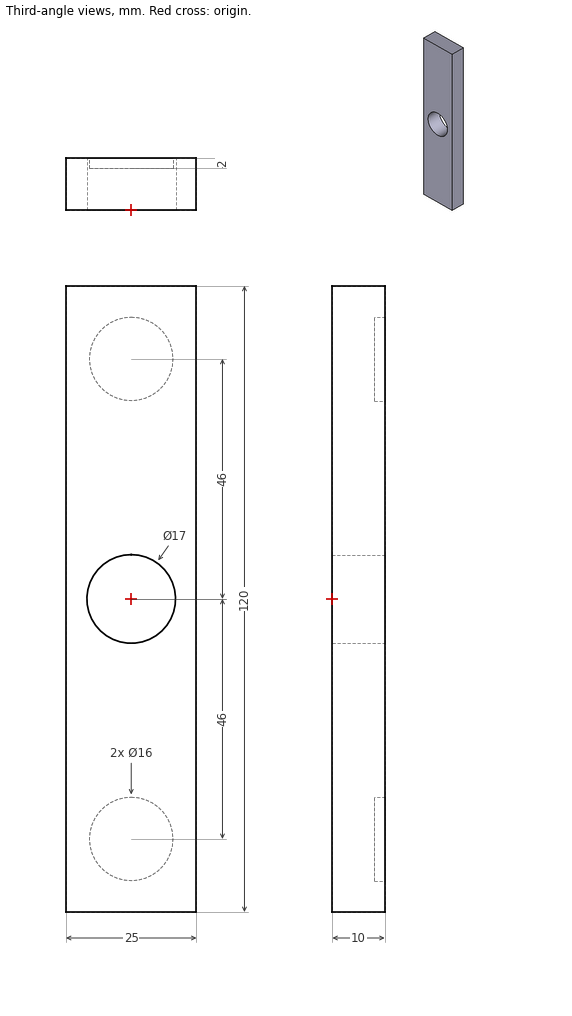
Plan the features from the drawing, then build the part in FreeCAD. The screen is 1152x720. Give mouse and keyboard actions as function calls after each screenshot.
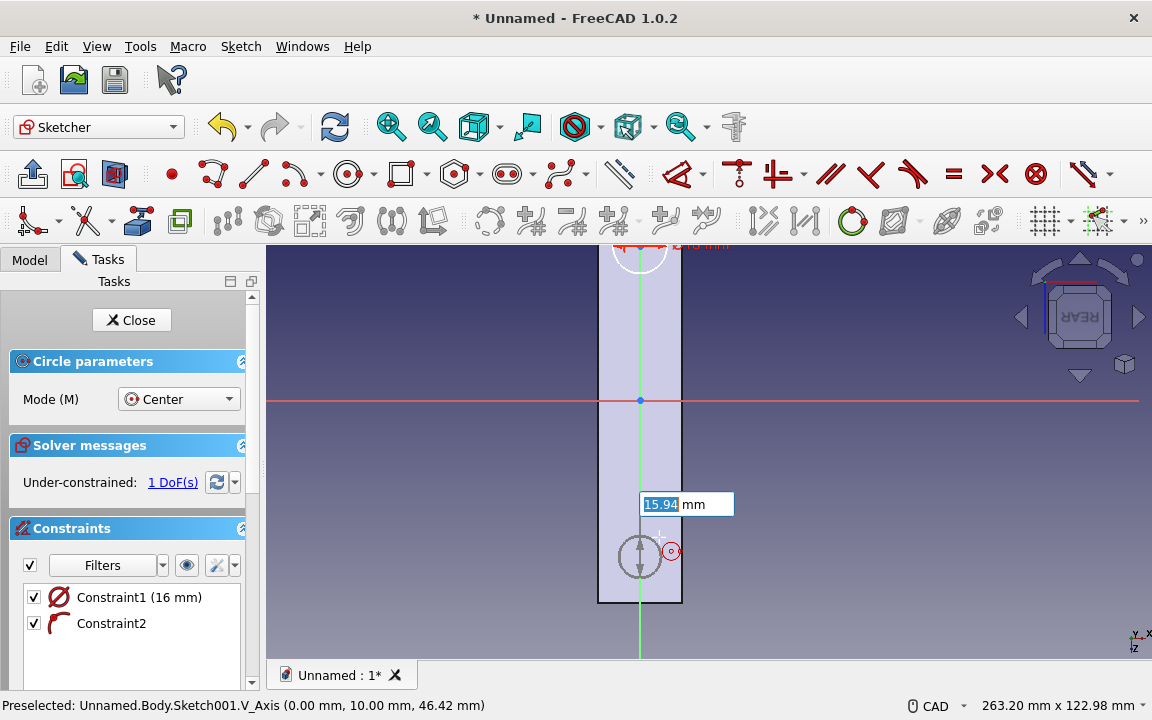
text(16)
key(Return)
key(Escape)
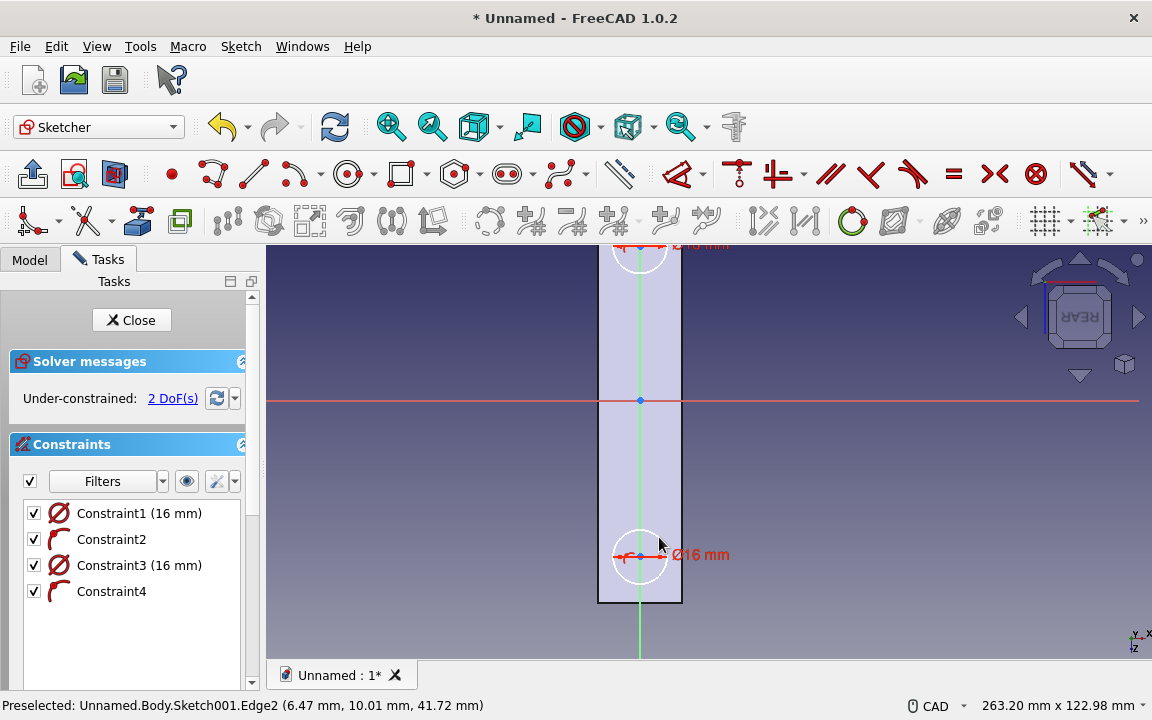
click(676, 174)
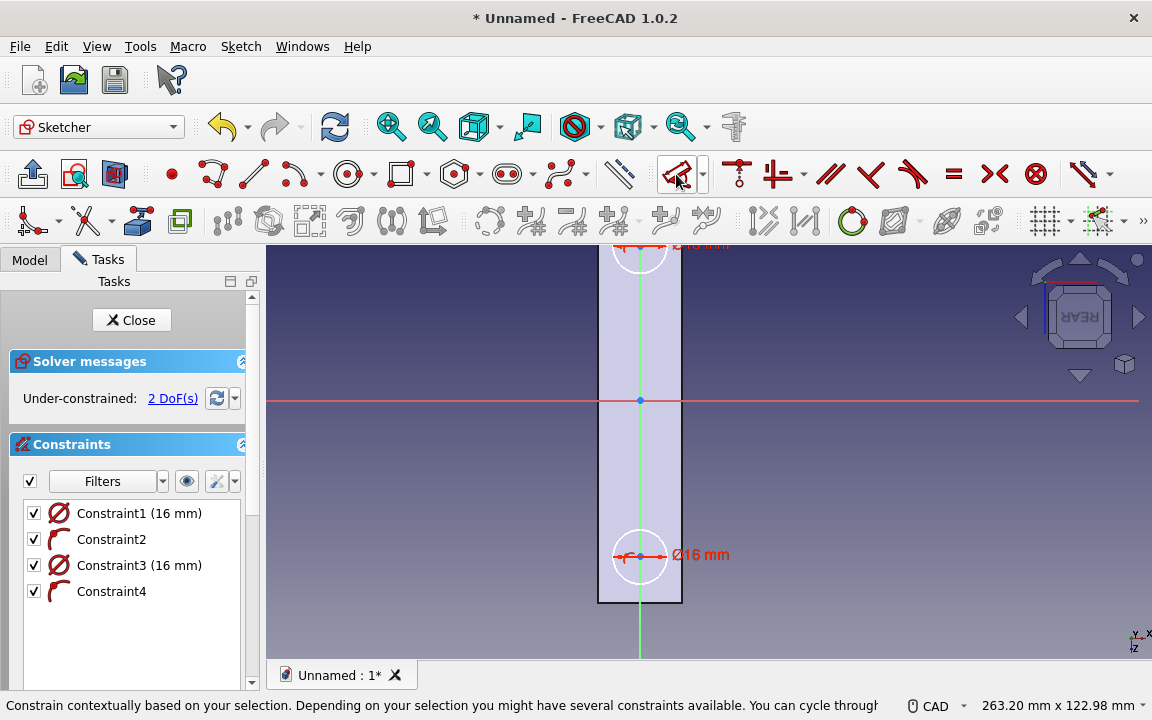
scroll(641, 556, down, 2)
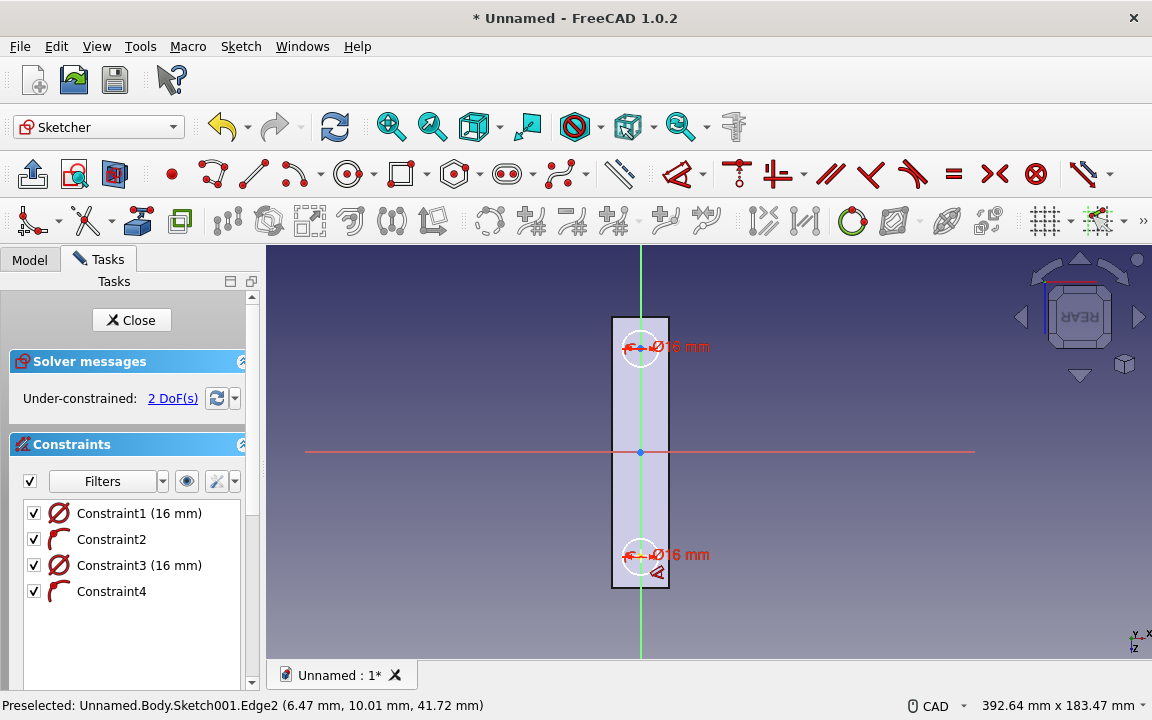
click(641, 349)
click(675, 400)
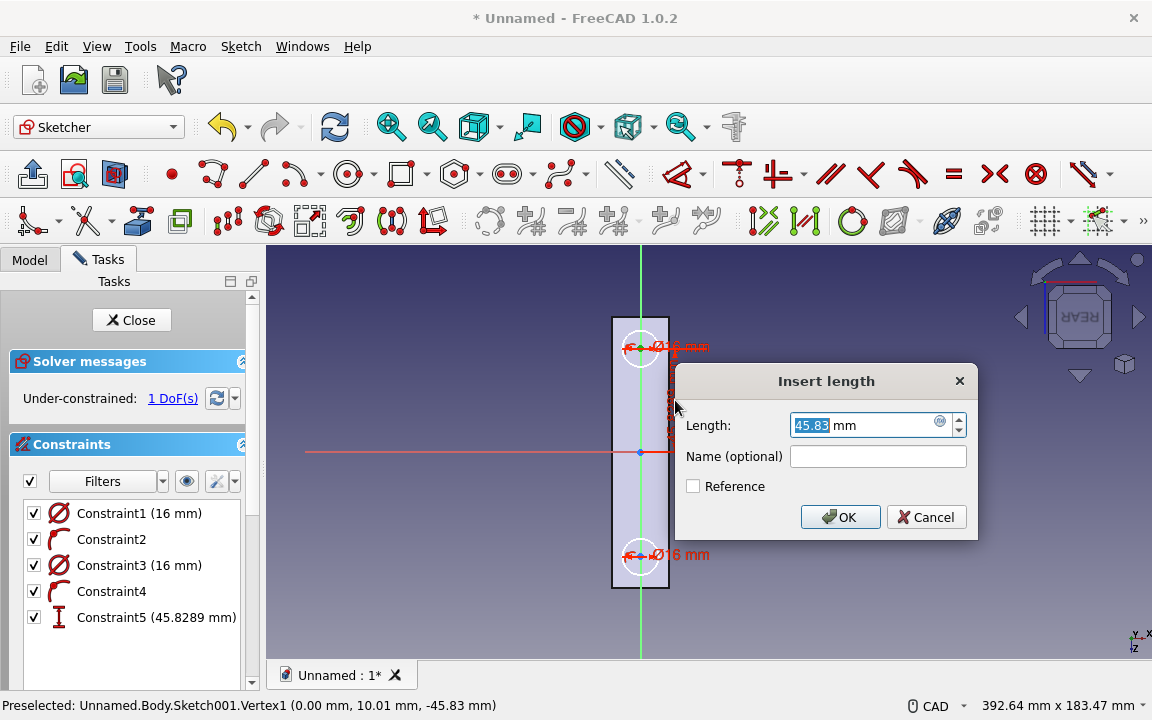
text(46)
key(Return)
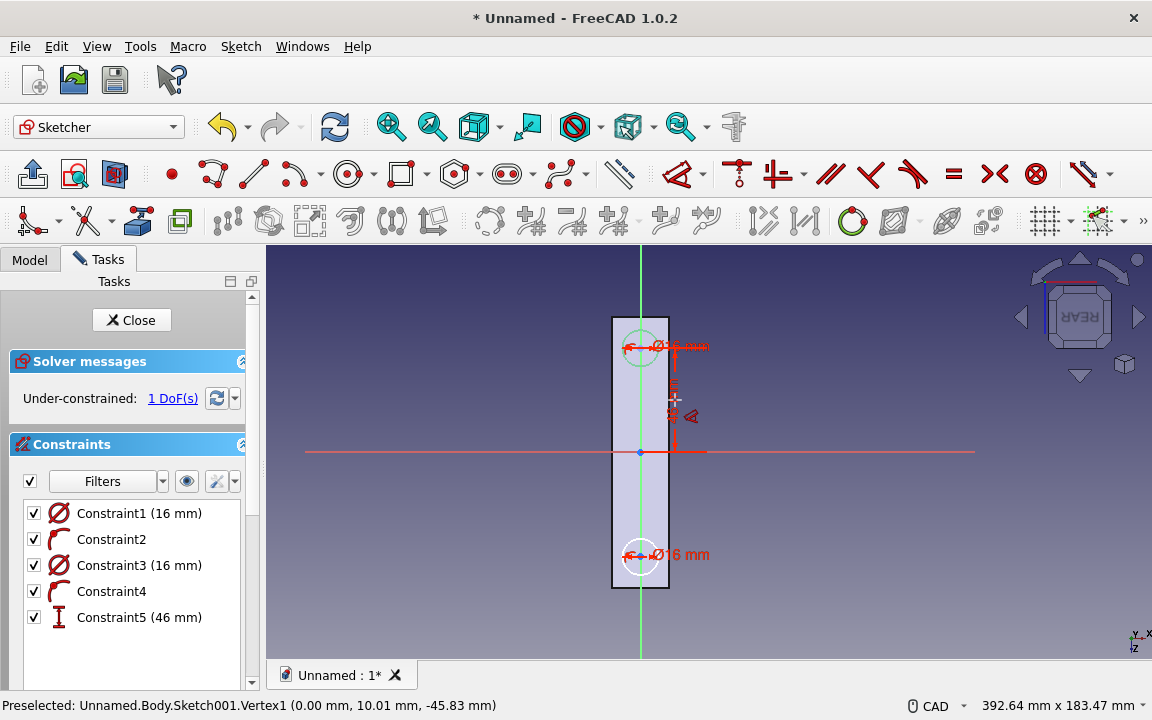
click(641, 557)
click(675, 505)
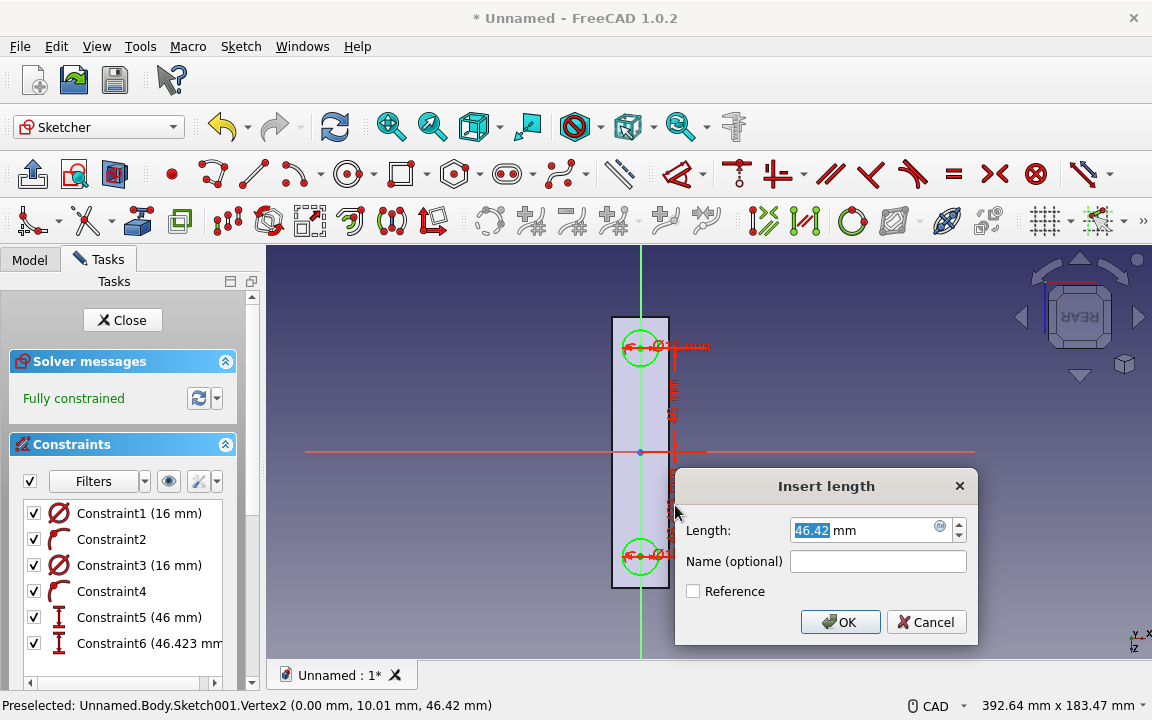
text(46)
key(Return)
key(Escape)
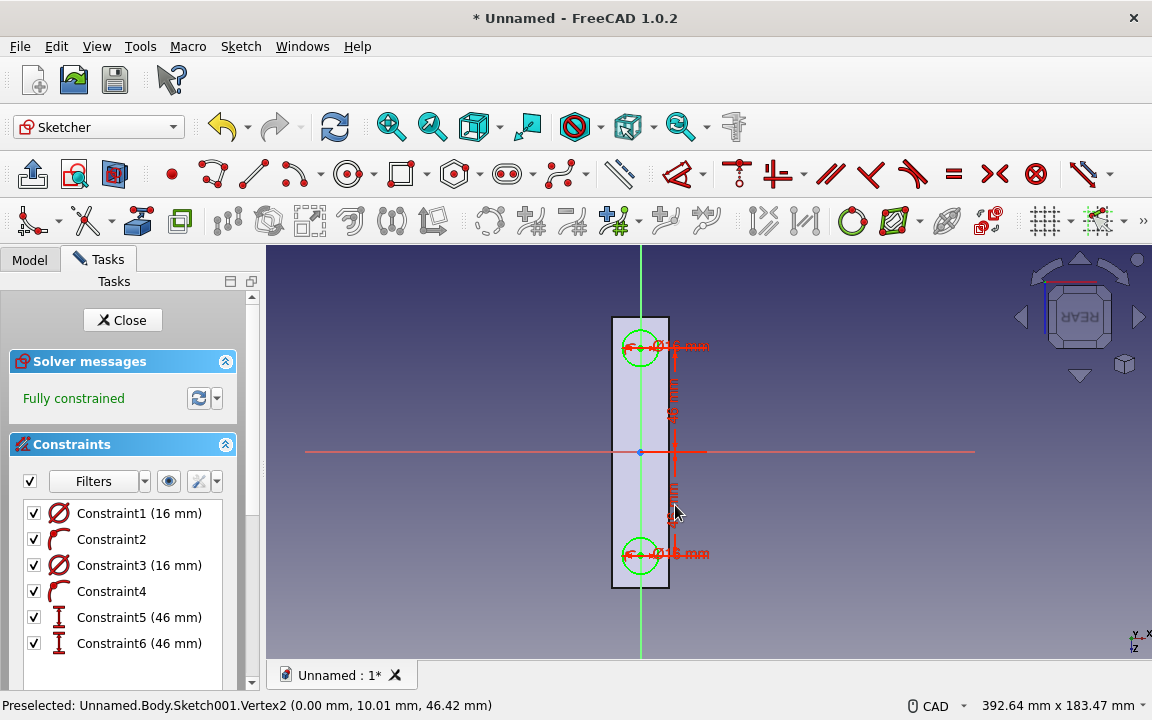
click(123, 320)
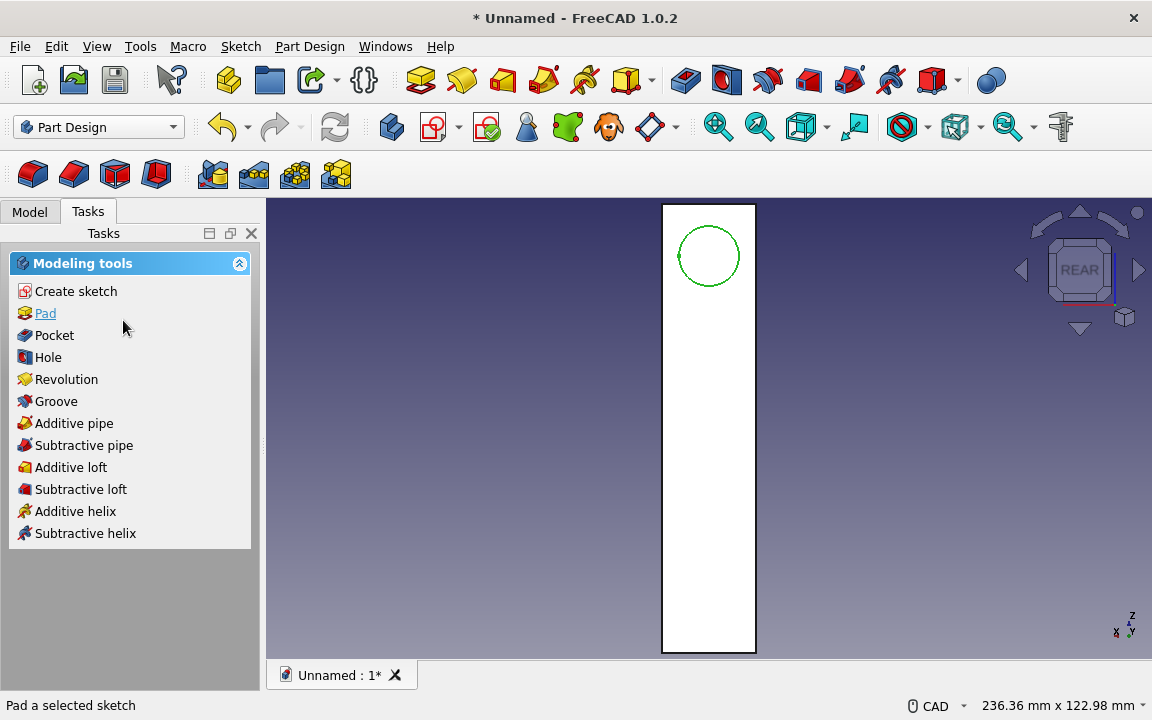
click(686, 80)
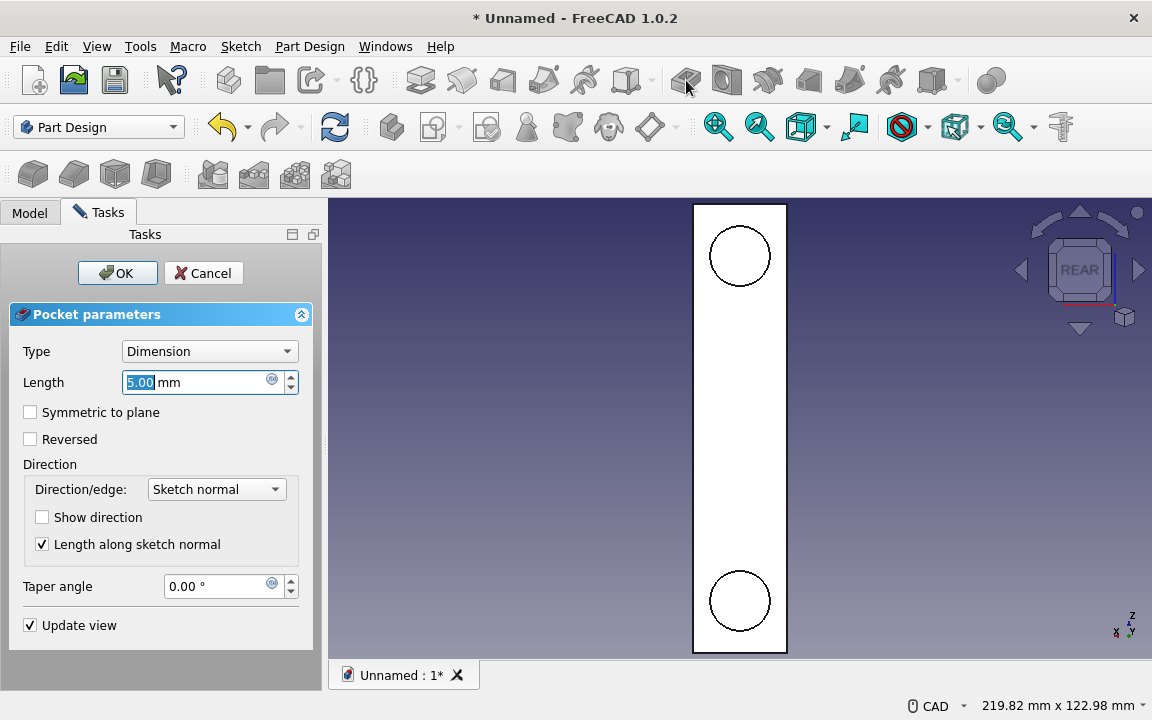
text(2)
key(Tab)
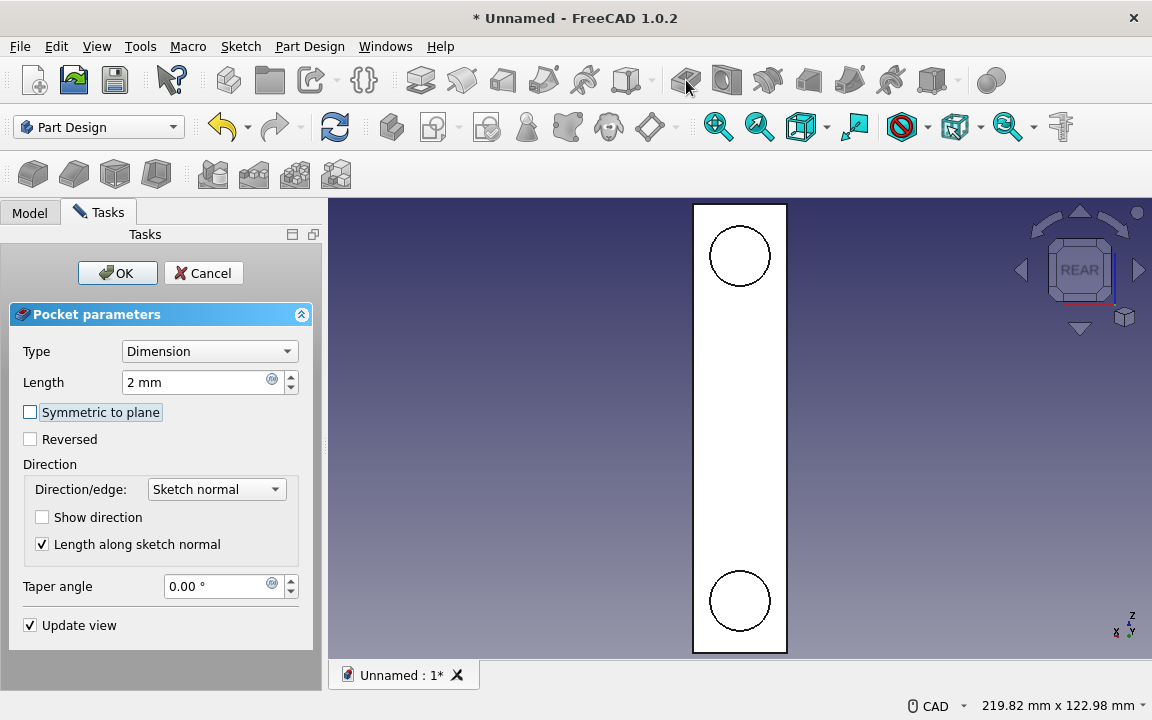
click(118, 273)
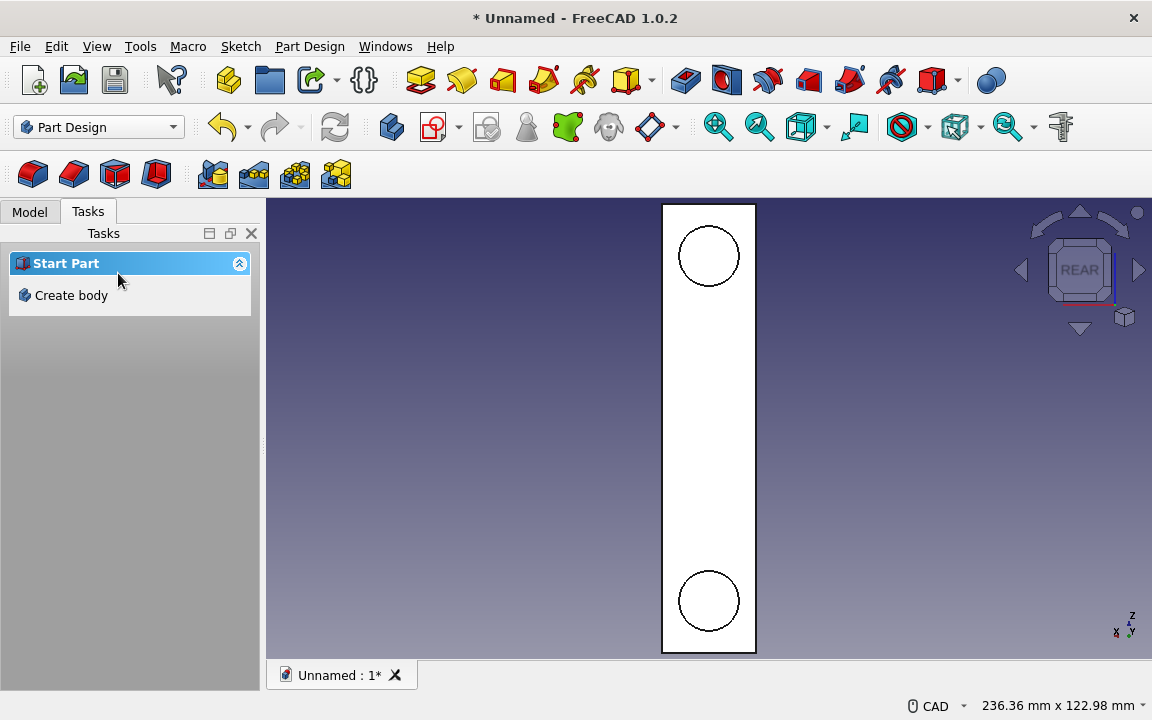
click(709, 363)